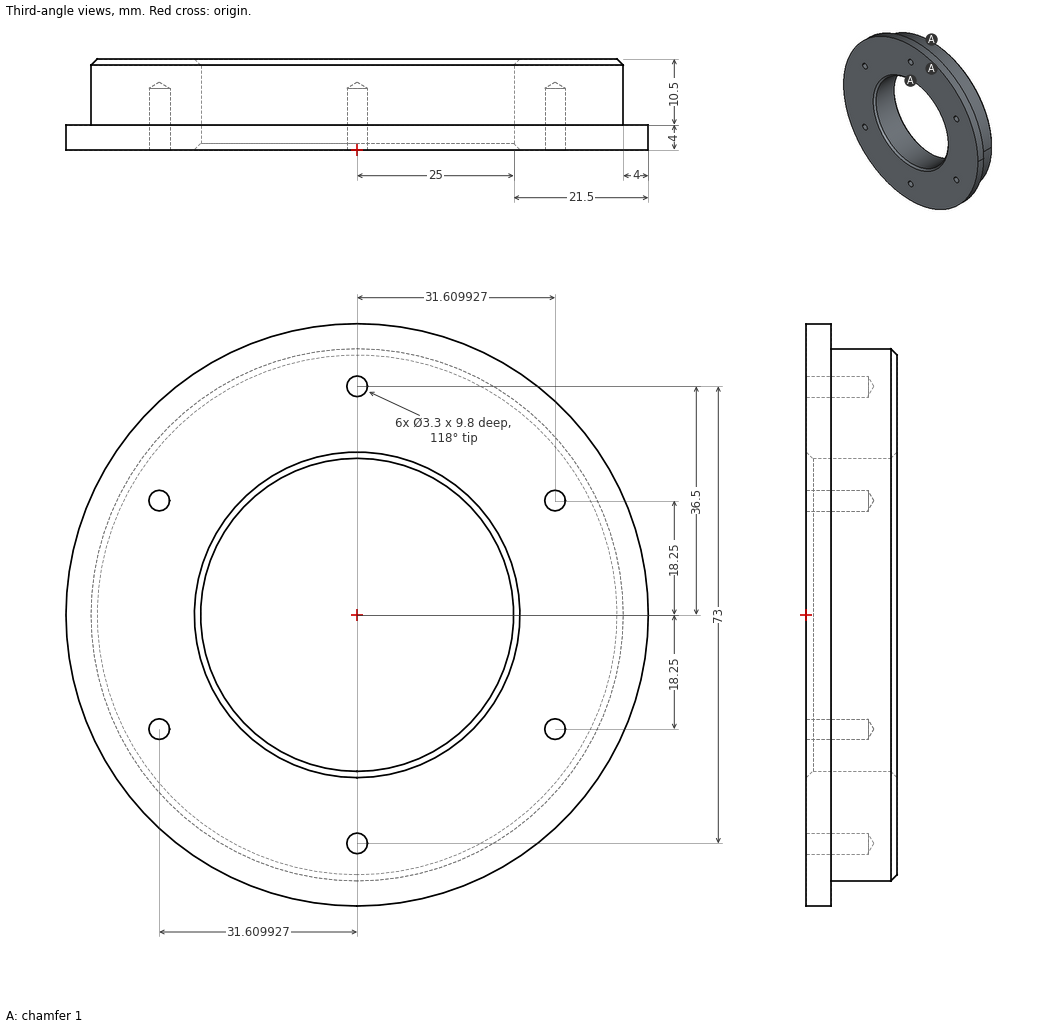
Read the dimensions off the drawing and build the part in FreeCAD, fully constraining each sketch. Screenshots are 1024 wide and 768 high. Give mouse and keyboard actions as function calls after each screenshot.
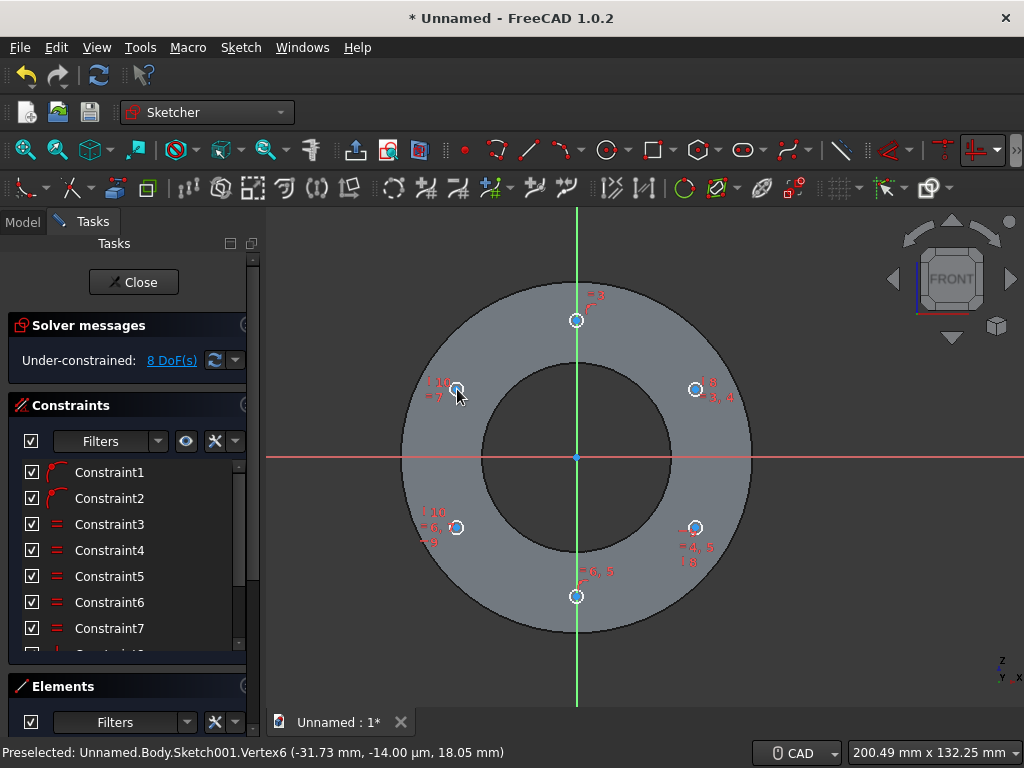
click(696, 389)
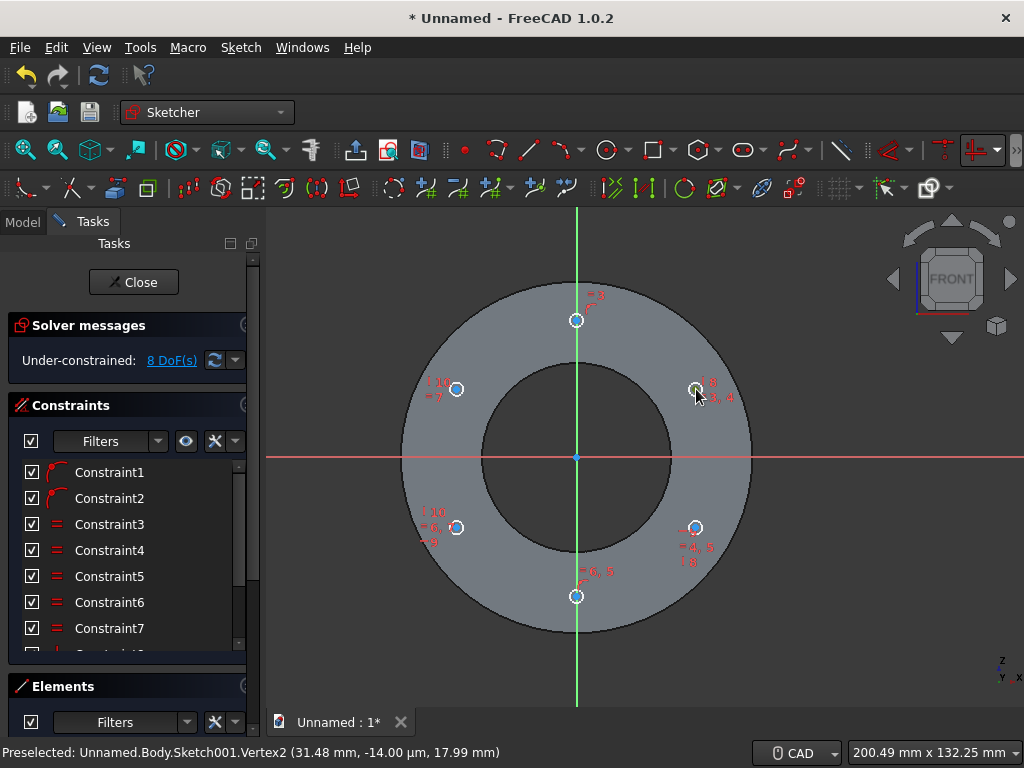
click(457, 389)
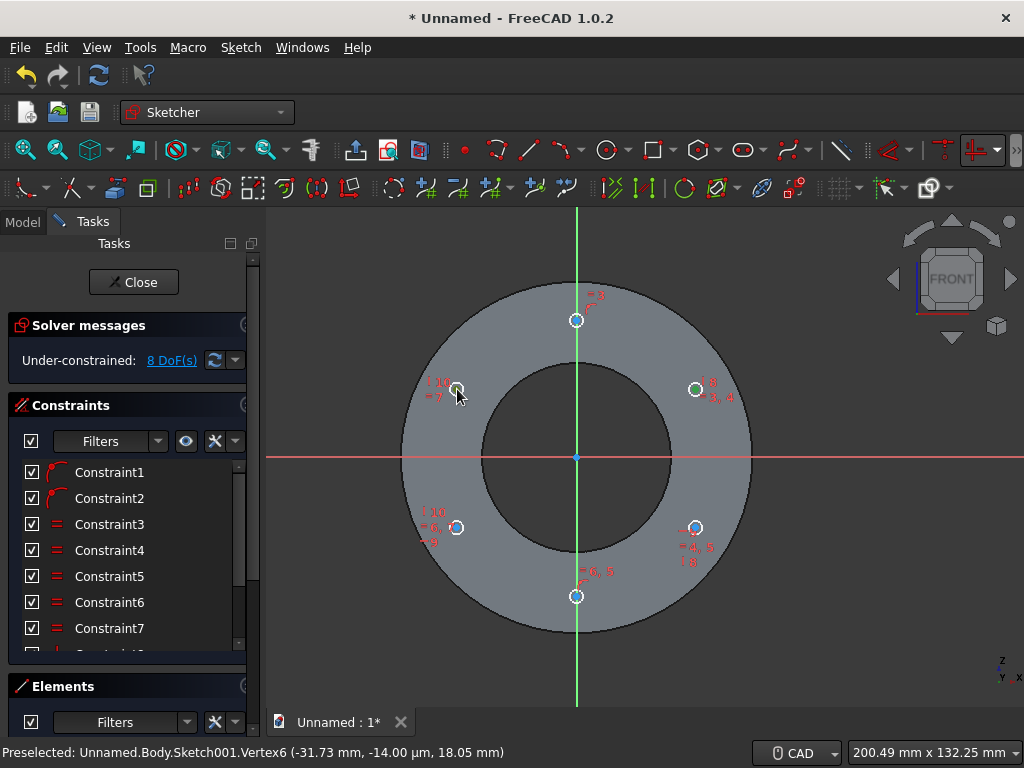
key(h)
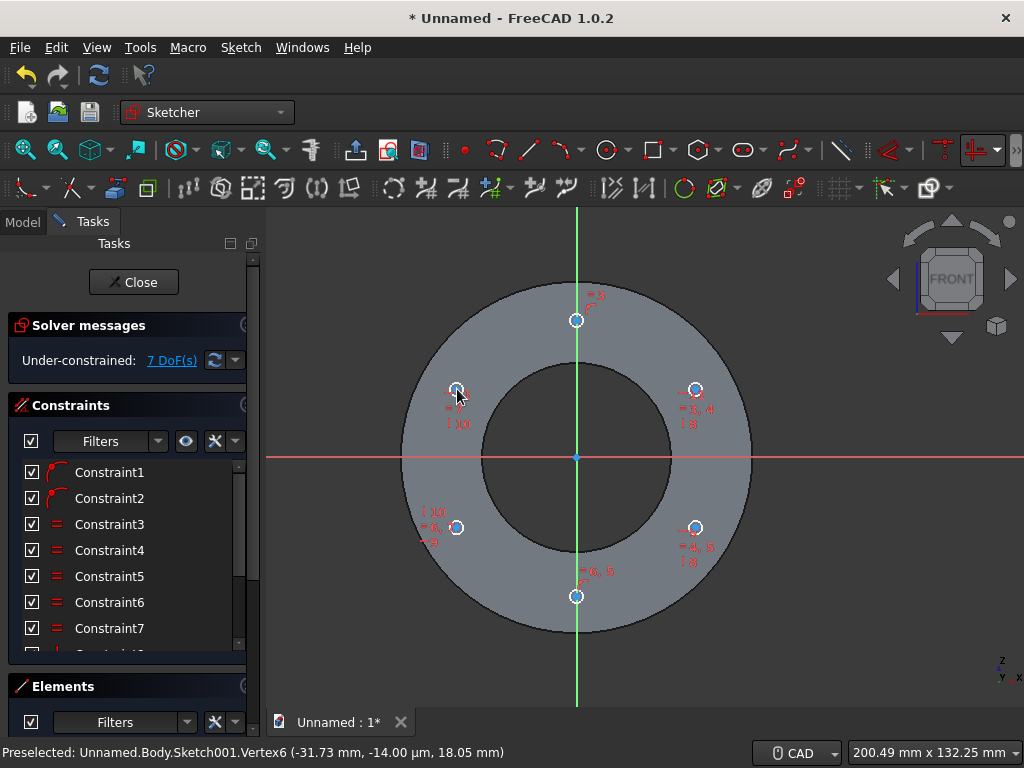
click(888, 150)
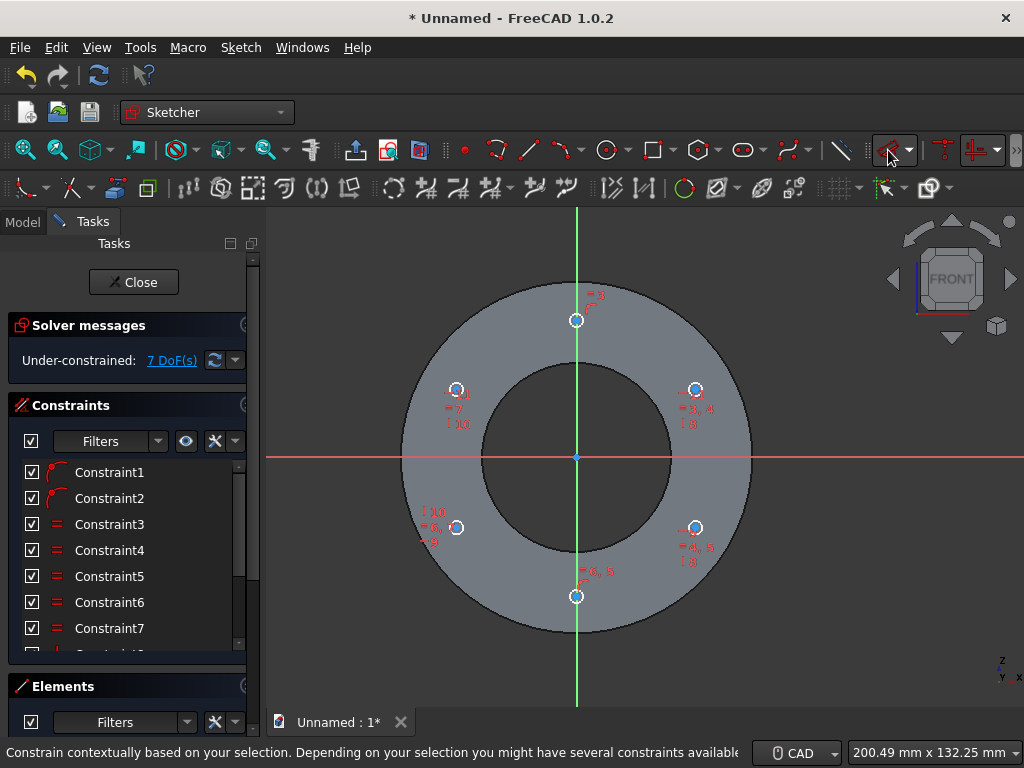
scroll(577, 314, up, 6)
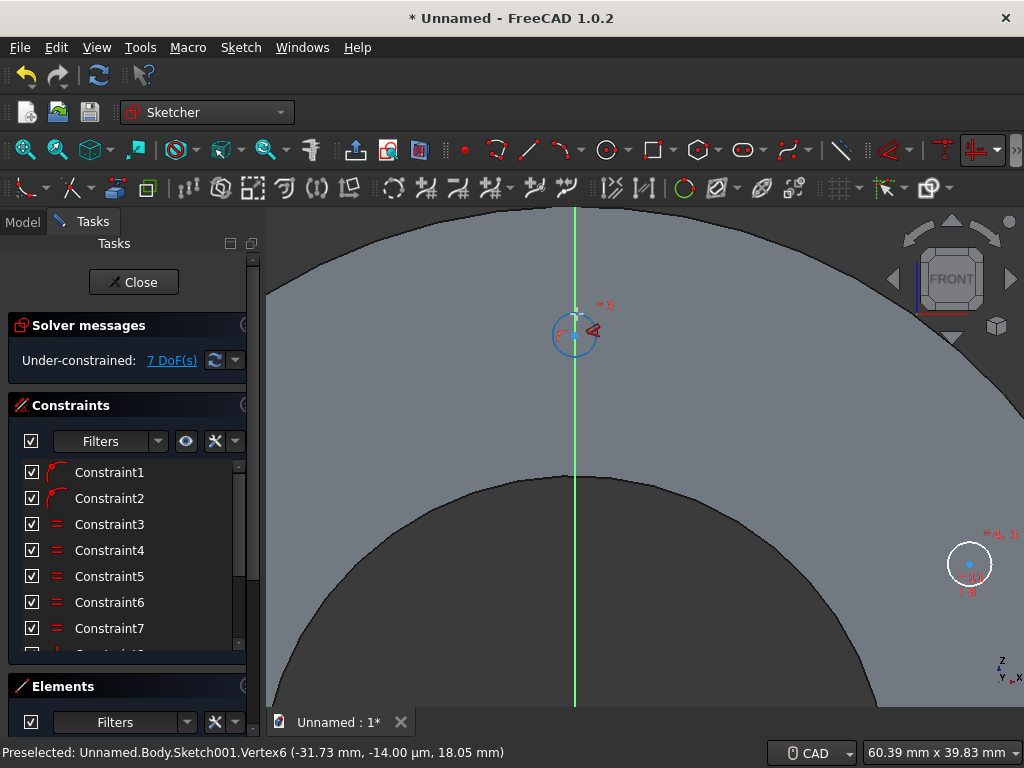
click(575, 313)
click(601, 288)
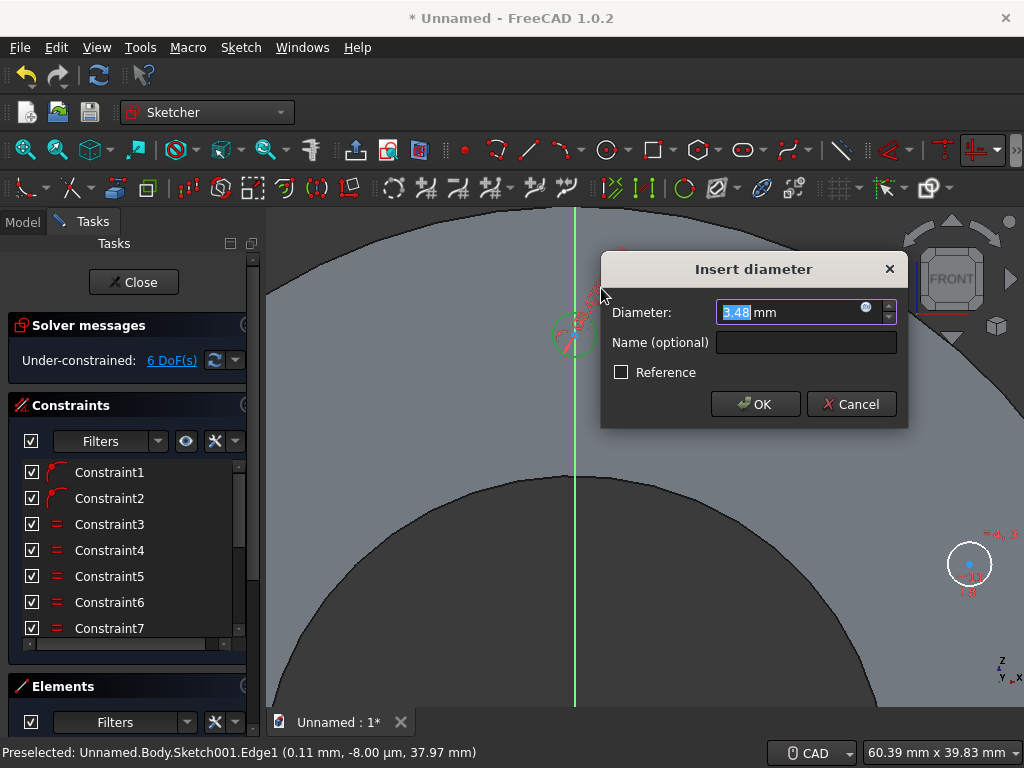
text(3.3)
key(Return)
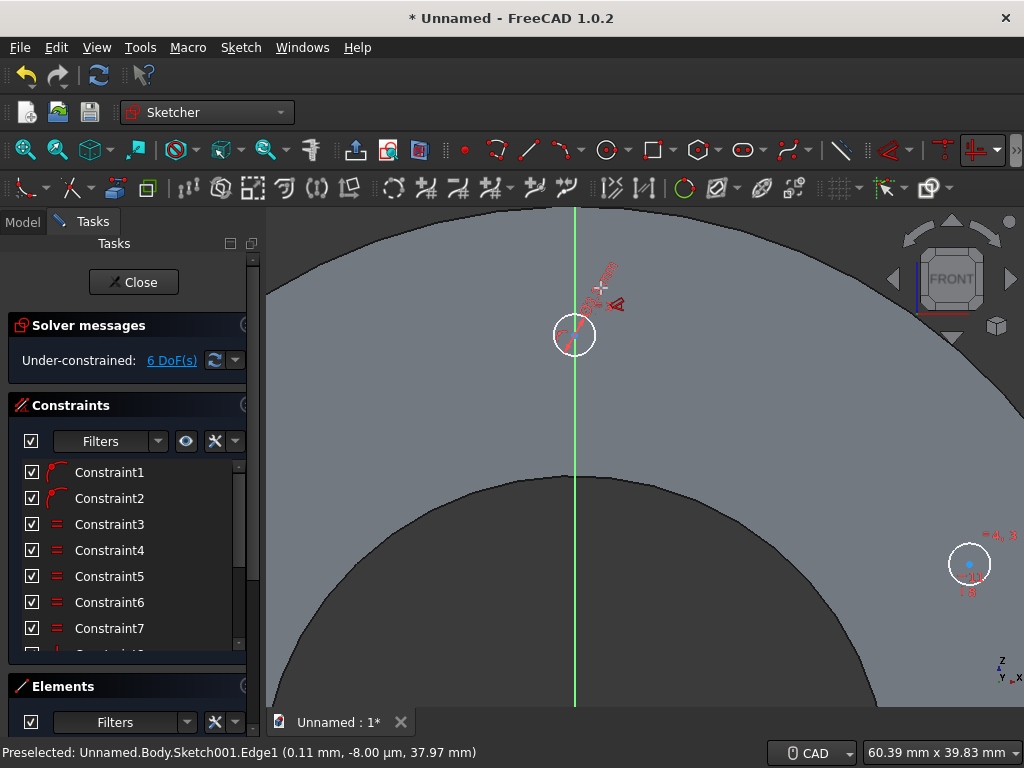
click(575, 335)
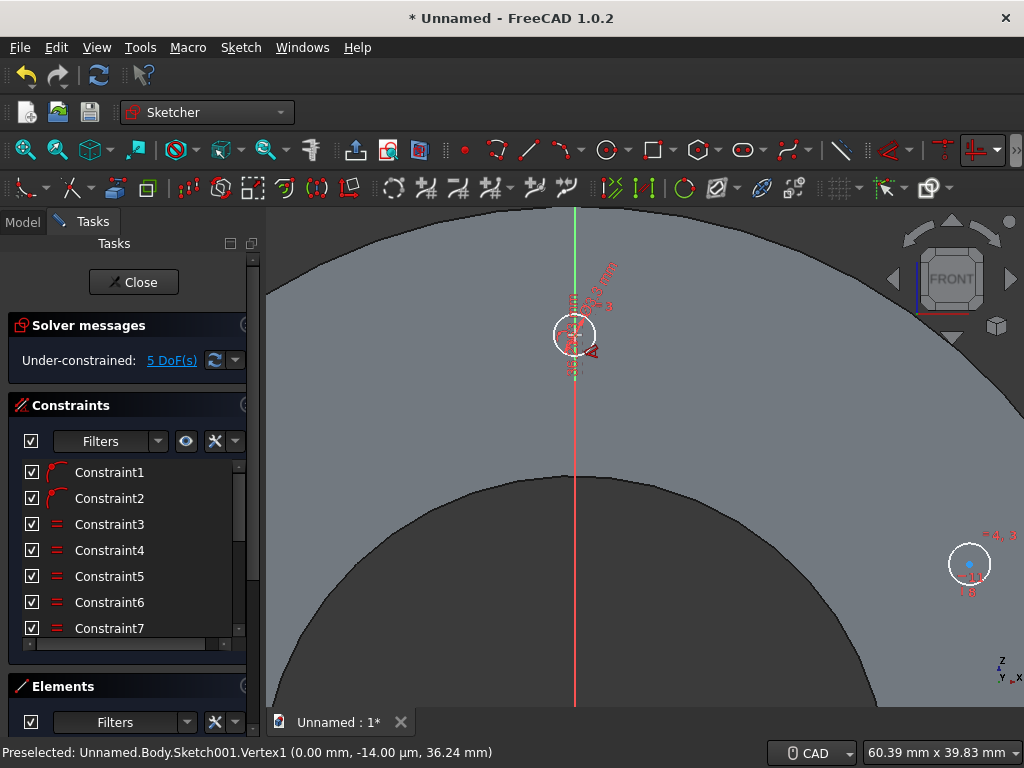
scroll(577, 314, down, 6)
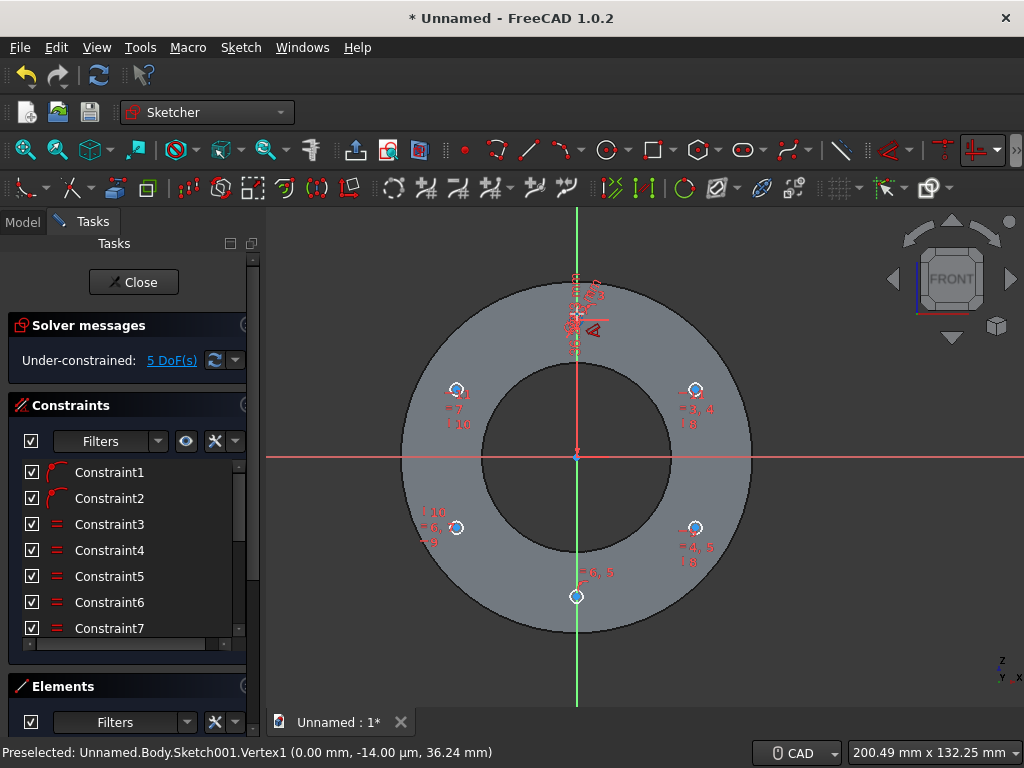
click(577, 597)
click(611, 395)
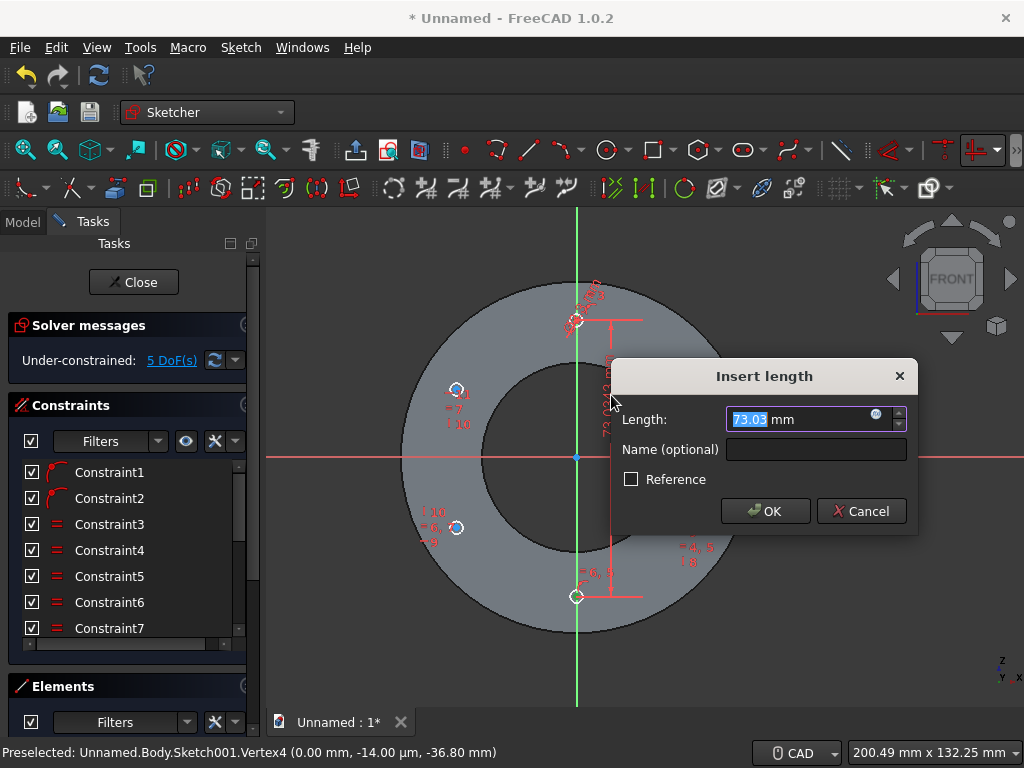
text(73)
key(Return)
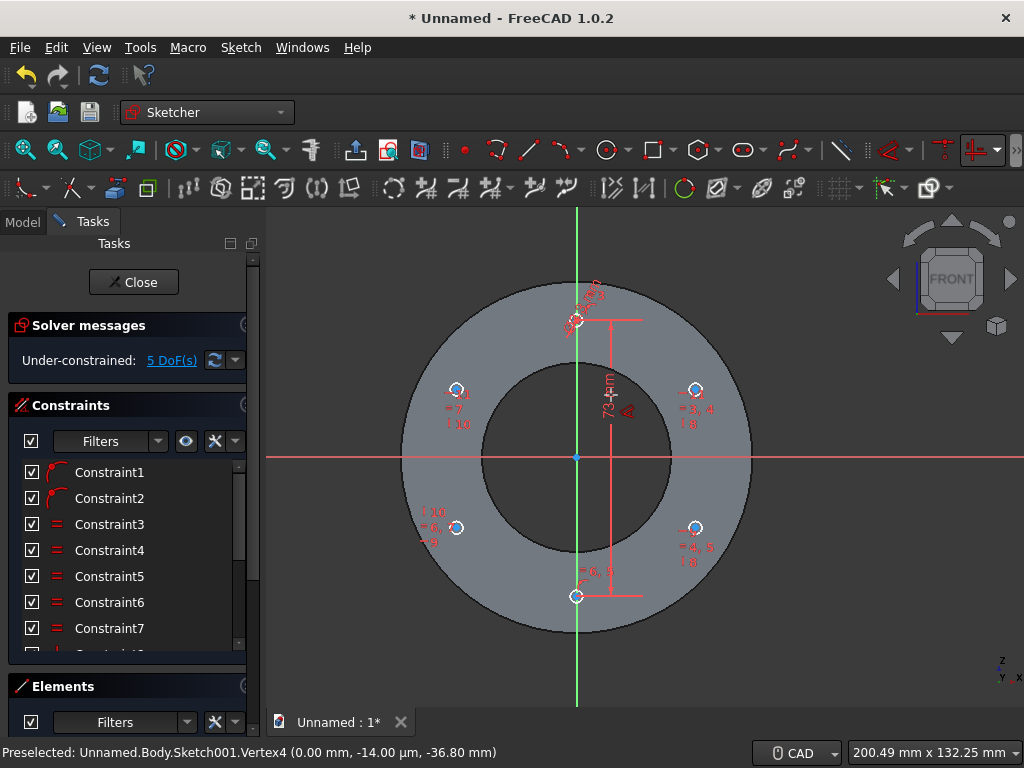
click(577, 320)
click(611, 357)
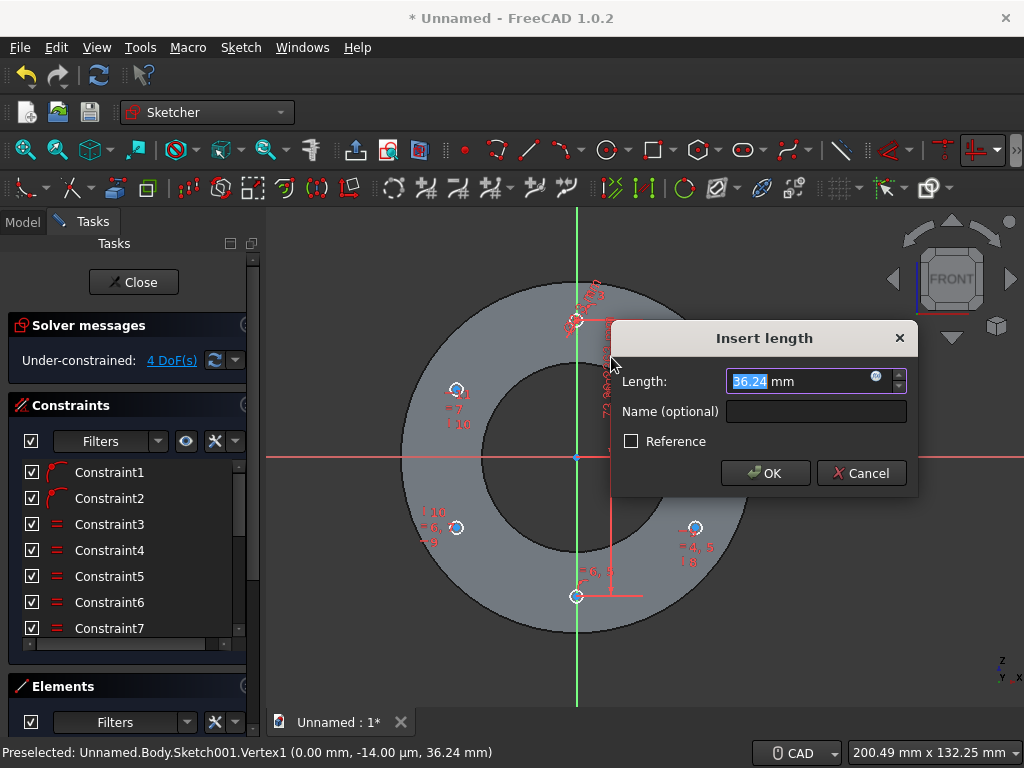
text(36.5)
key(Return)